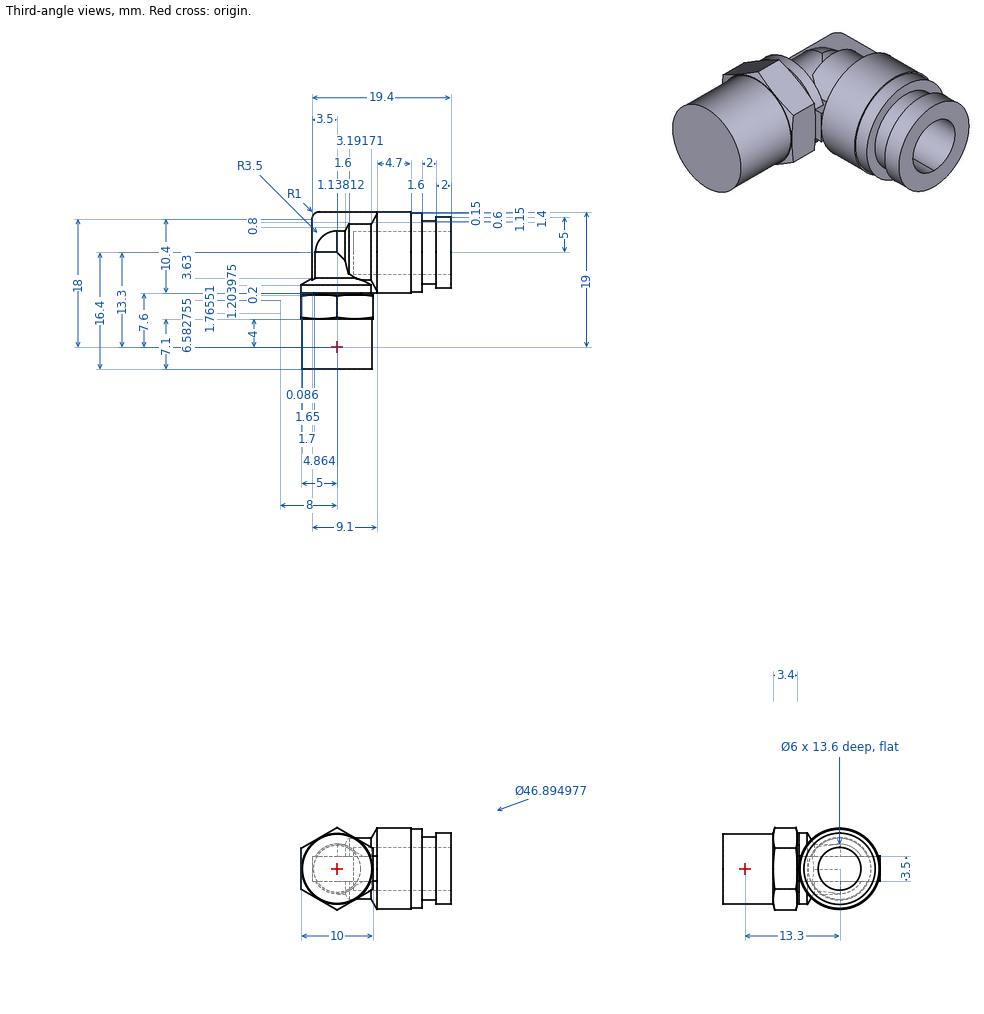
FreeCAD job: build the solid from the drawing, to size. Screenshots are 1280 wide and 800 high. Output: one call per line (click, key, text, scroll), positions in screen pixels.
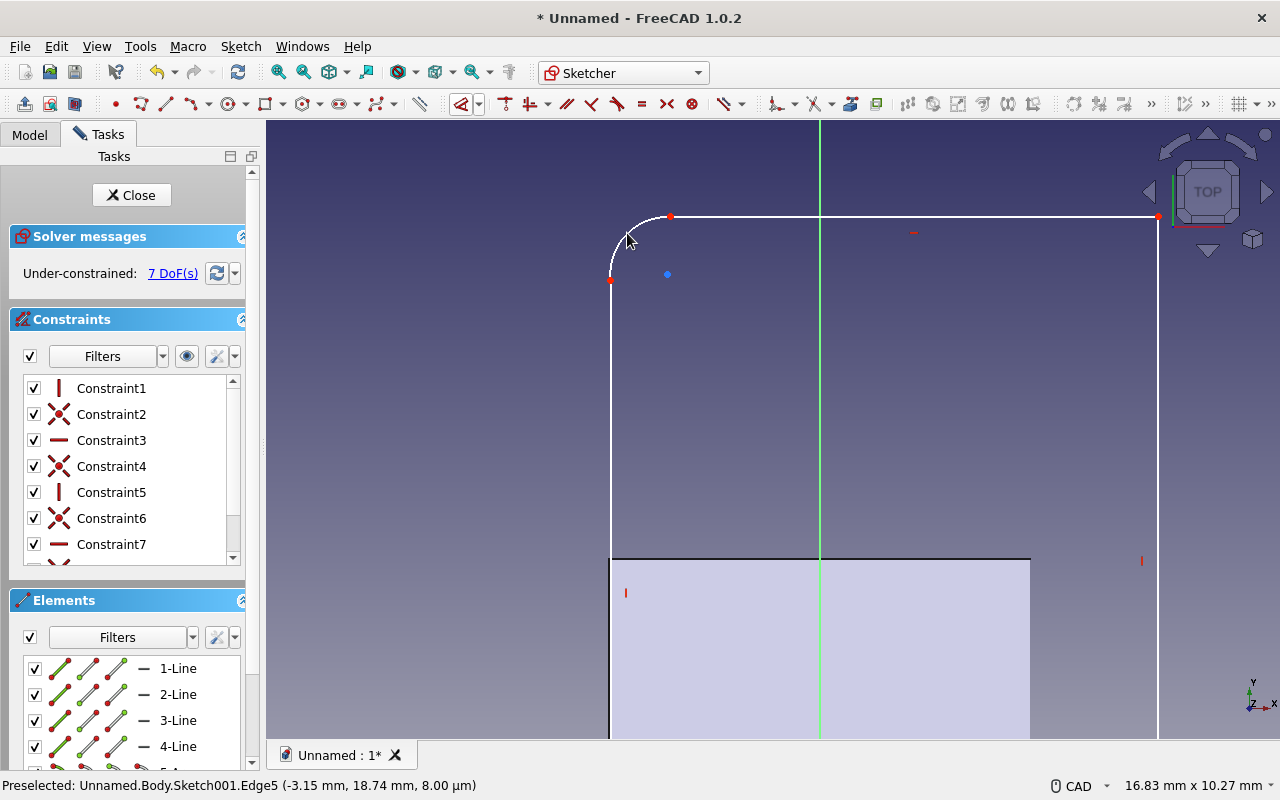
click(611, 467)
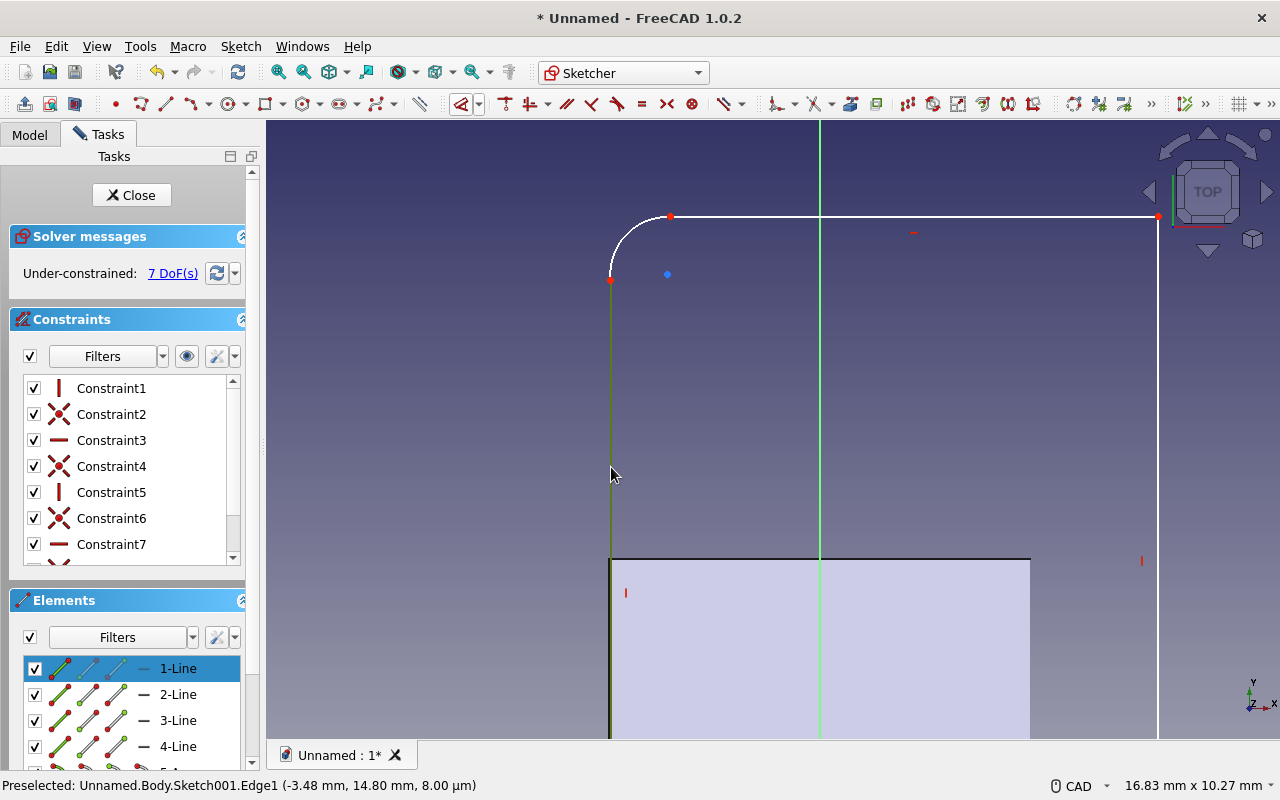
click(642, 223)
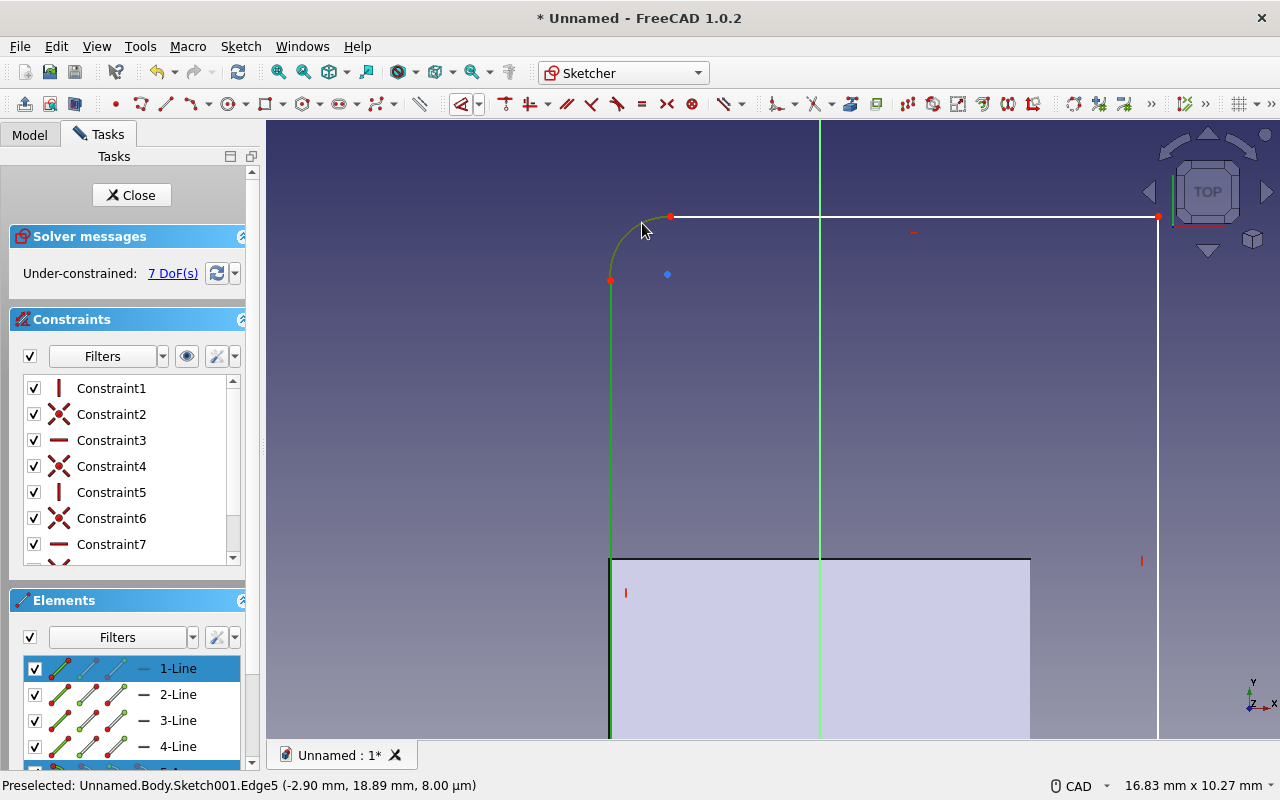
key(t)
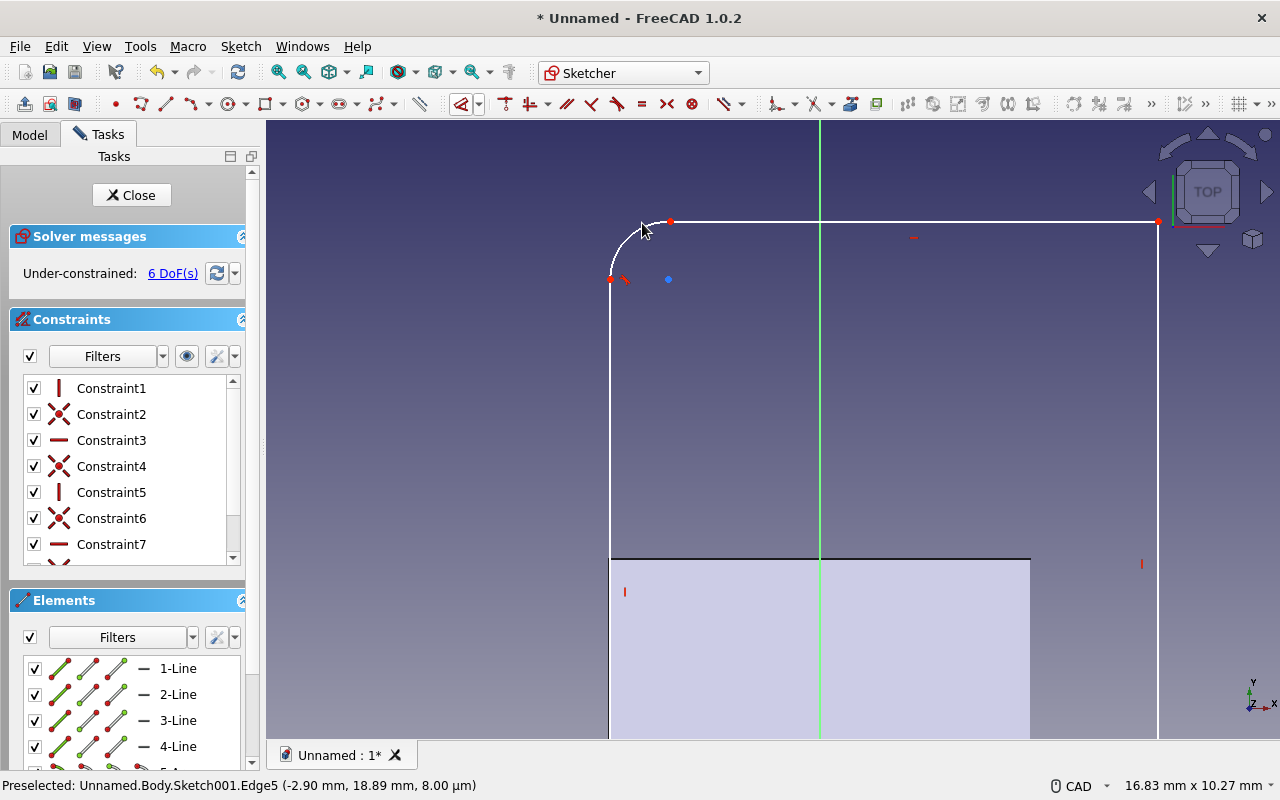
click(1012, 222)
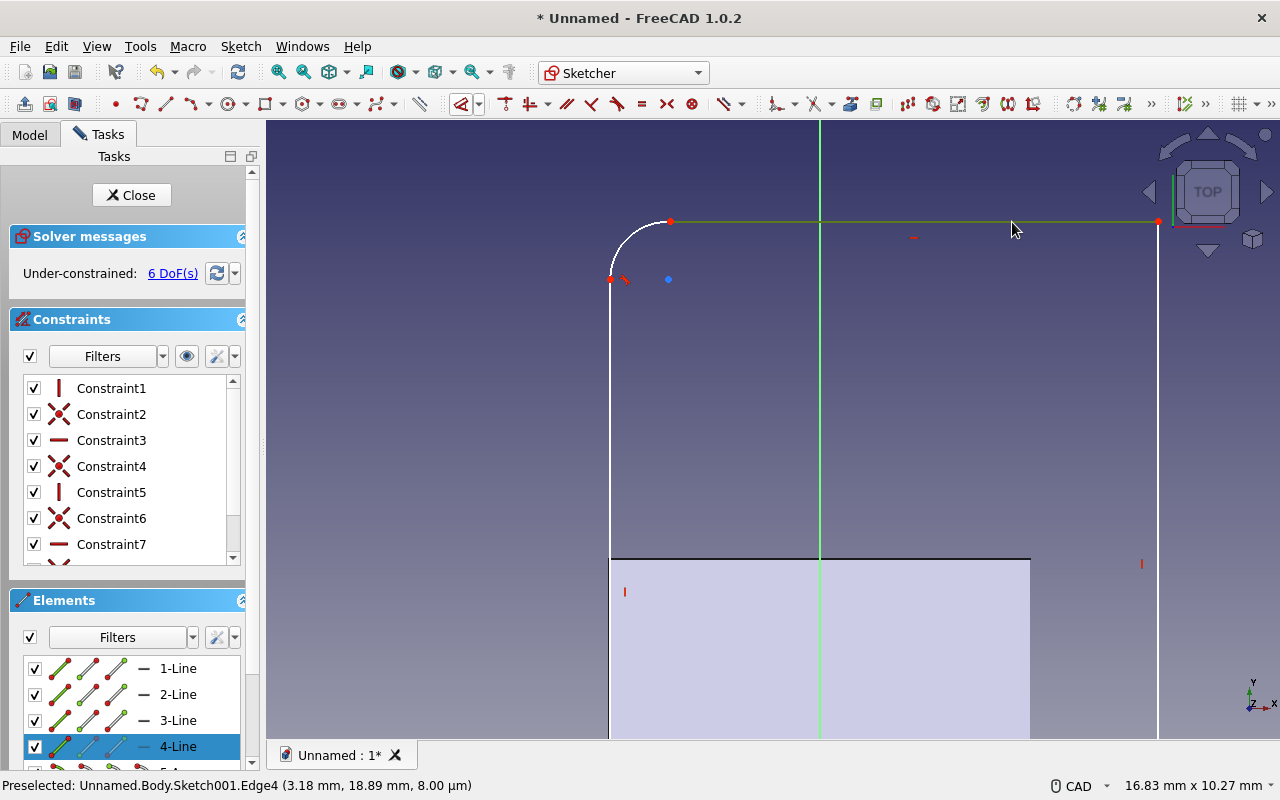
click(643, 227)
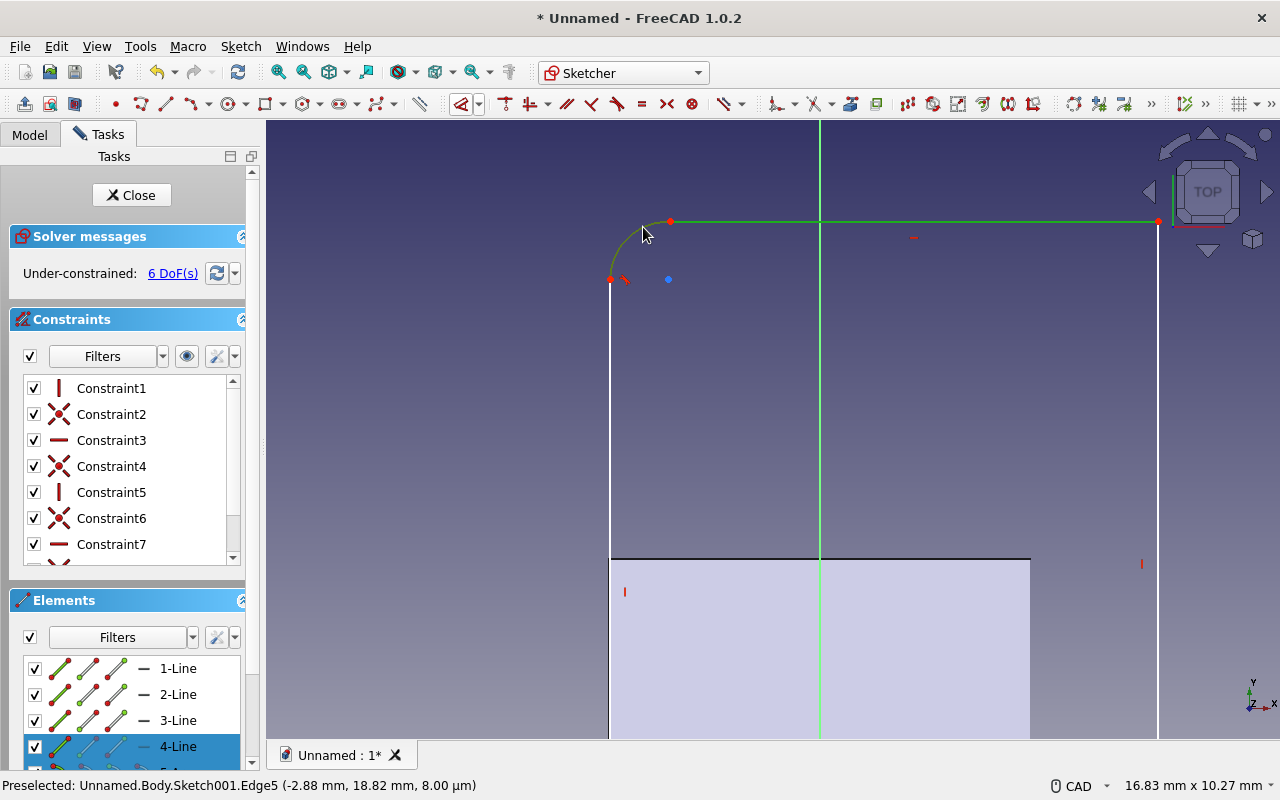
click(617, 104)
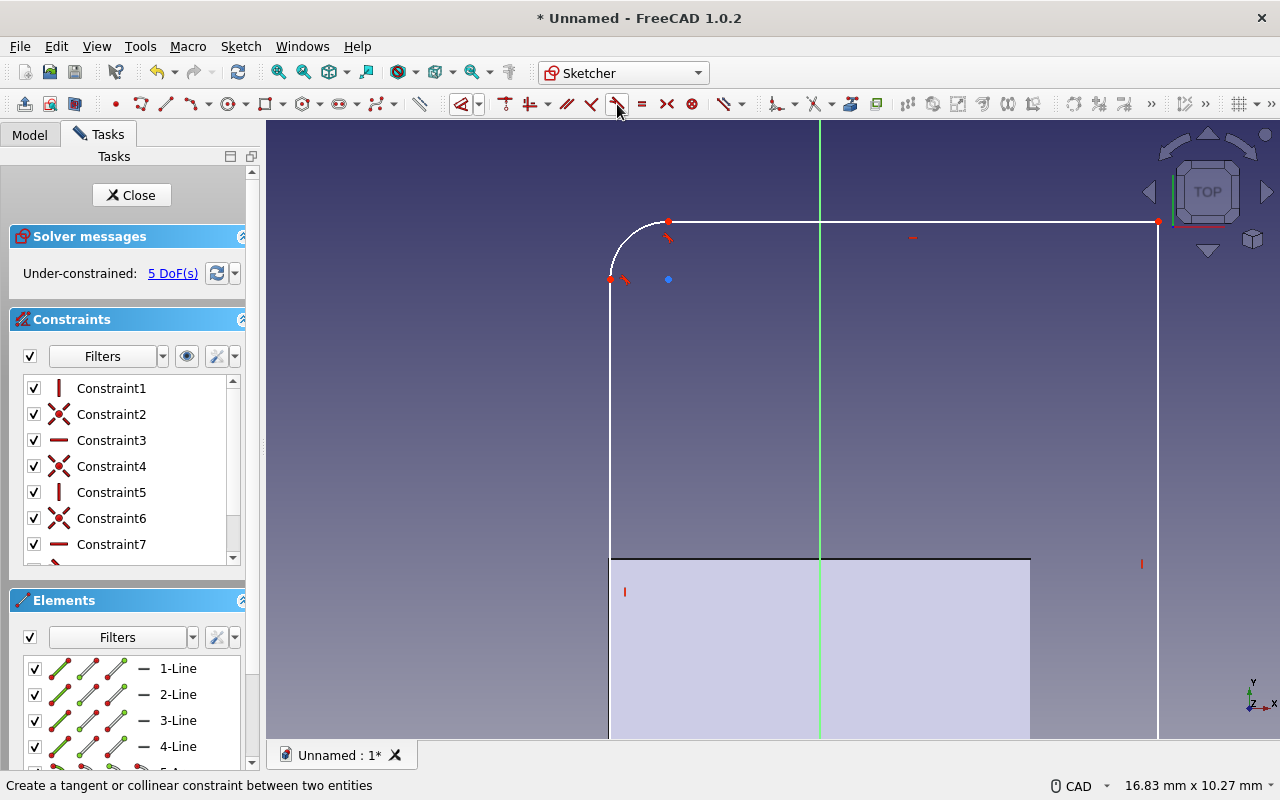
click(642, 228)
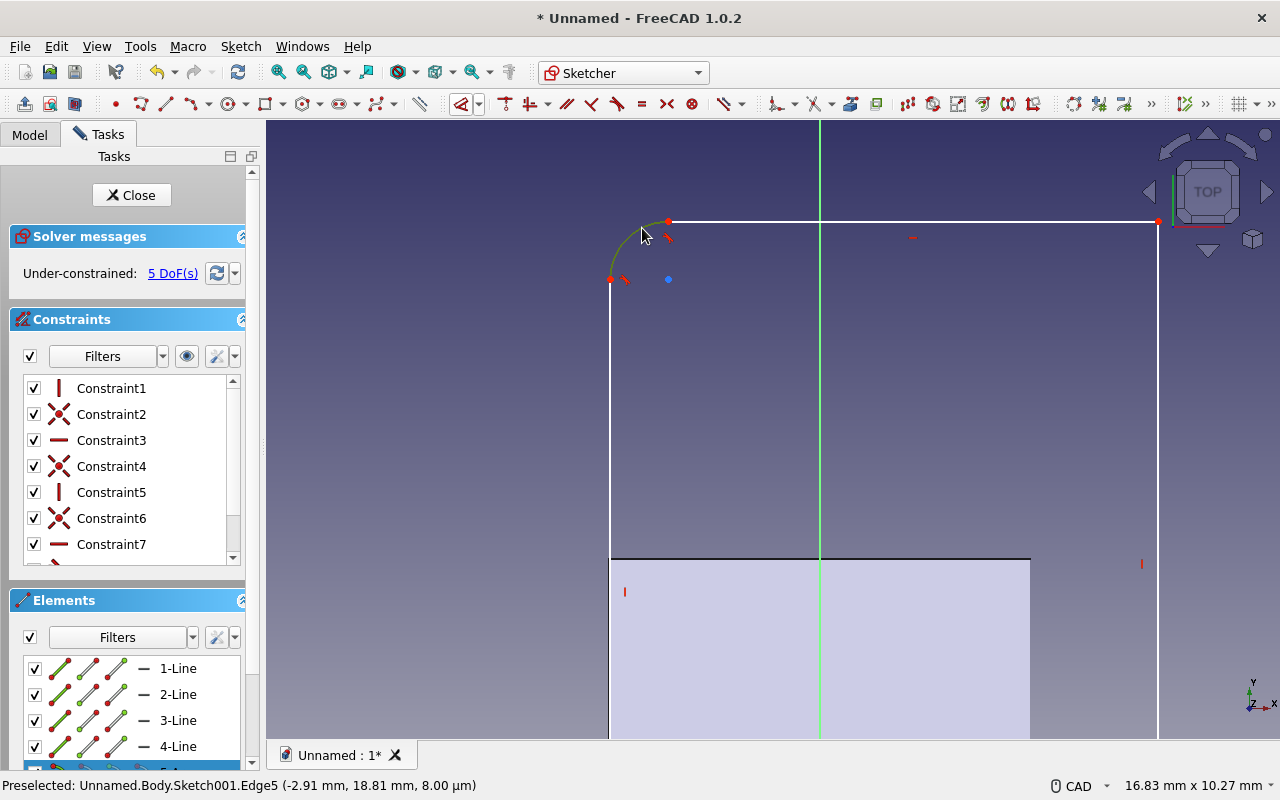
click(478, 104)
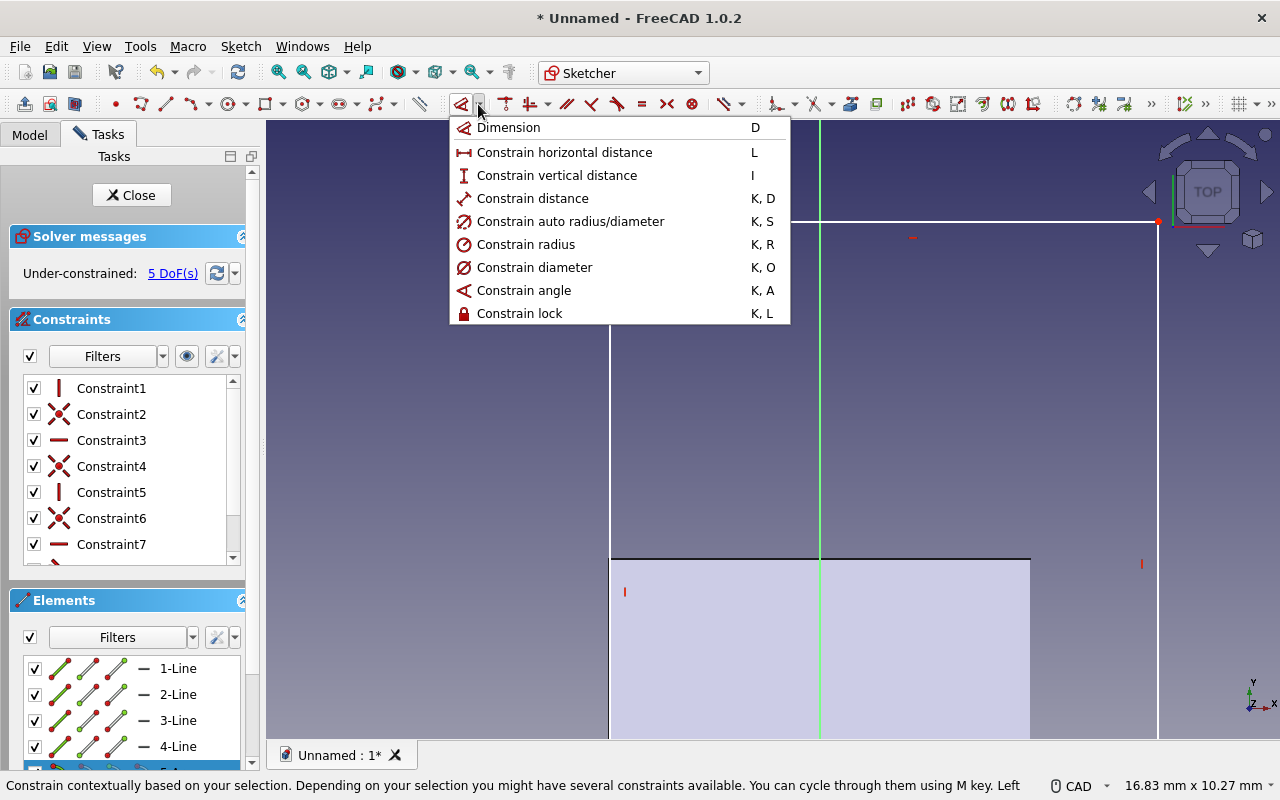
click(620, 244)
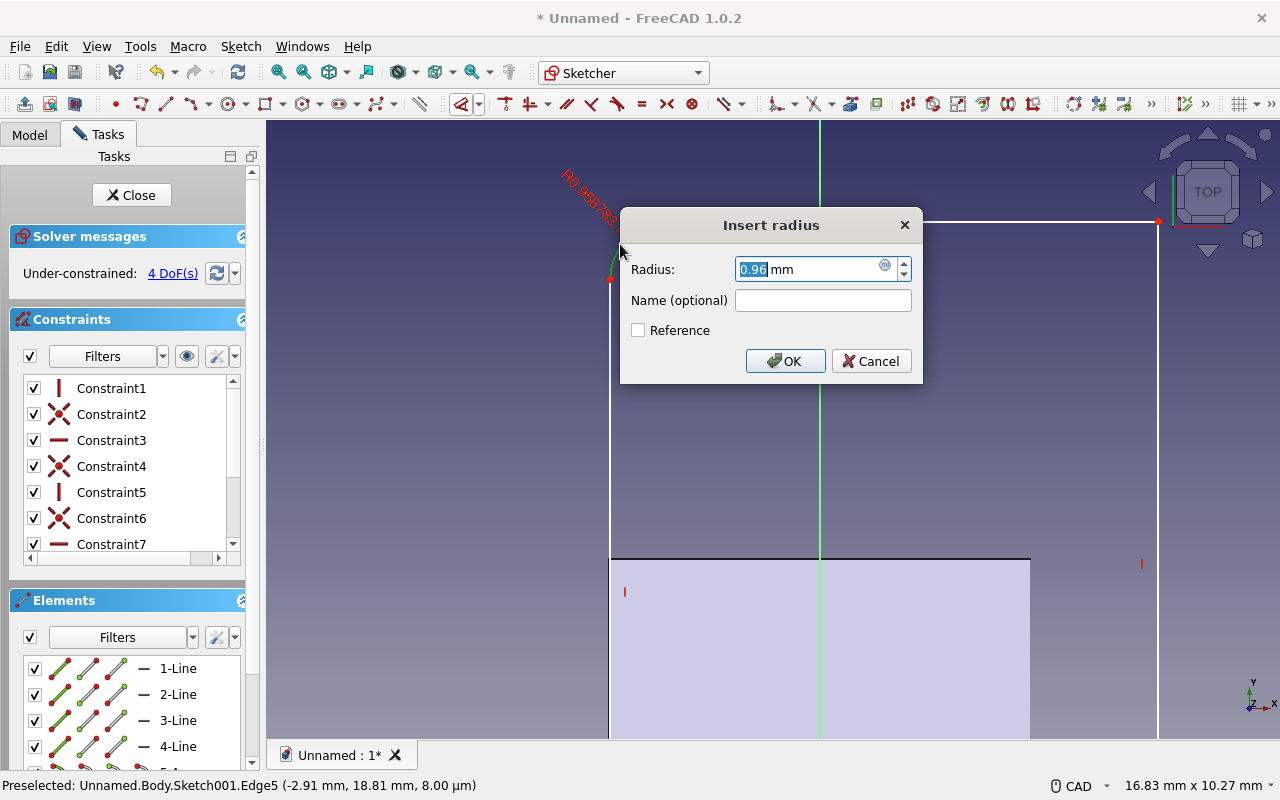
text(1)
key(Return)